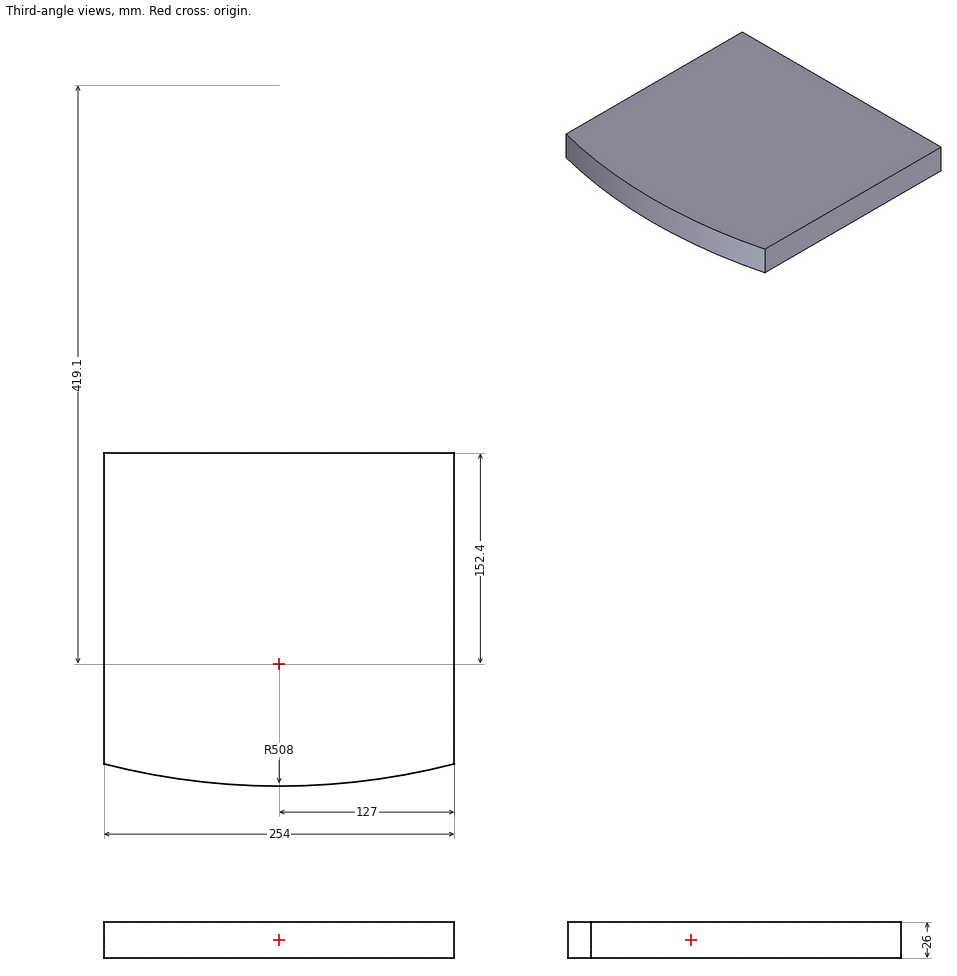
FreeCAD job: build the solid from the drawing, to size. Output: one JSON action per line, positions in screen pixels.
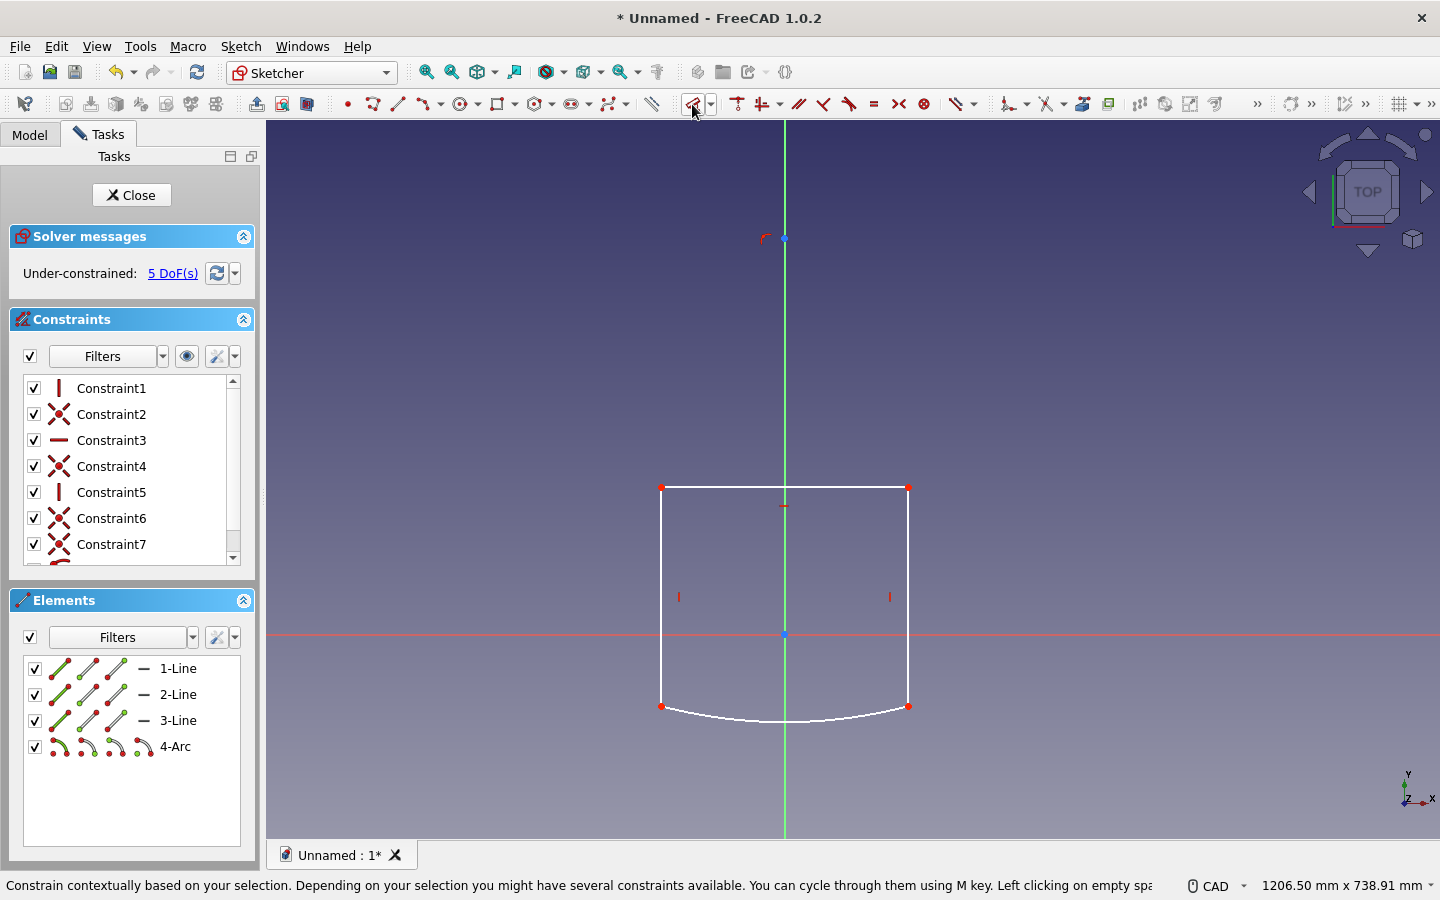
{"action": "left_click", "coordinate": [735, 720]}
{"action": "left_click", "coordinate": [732, 752]}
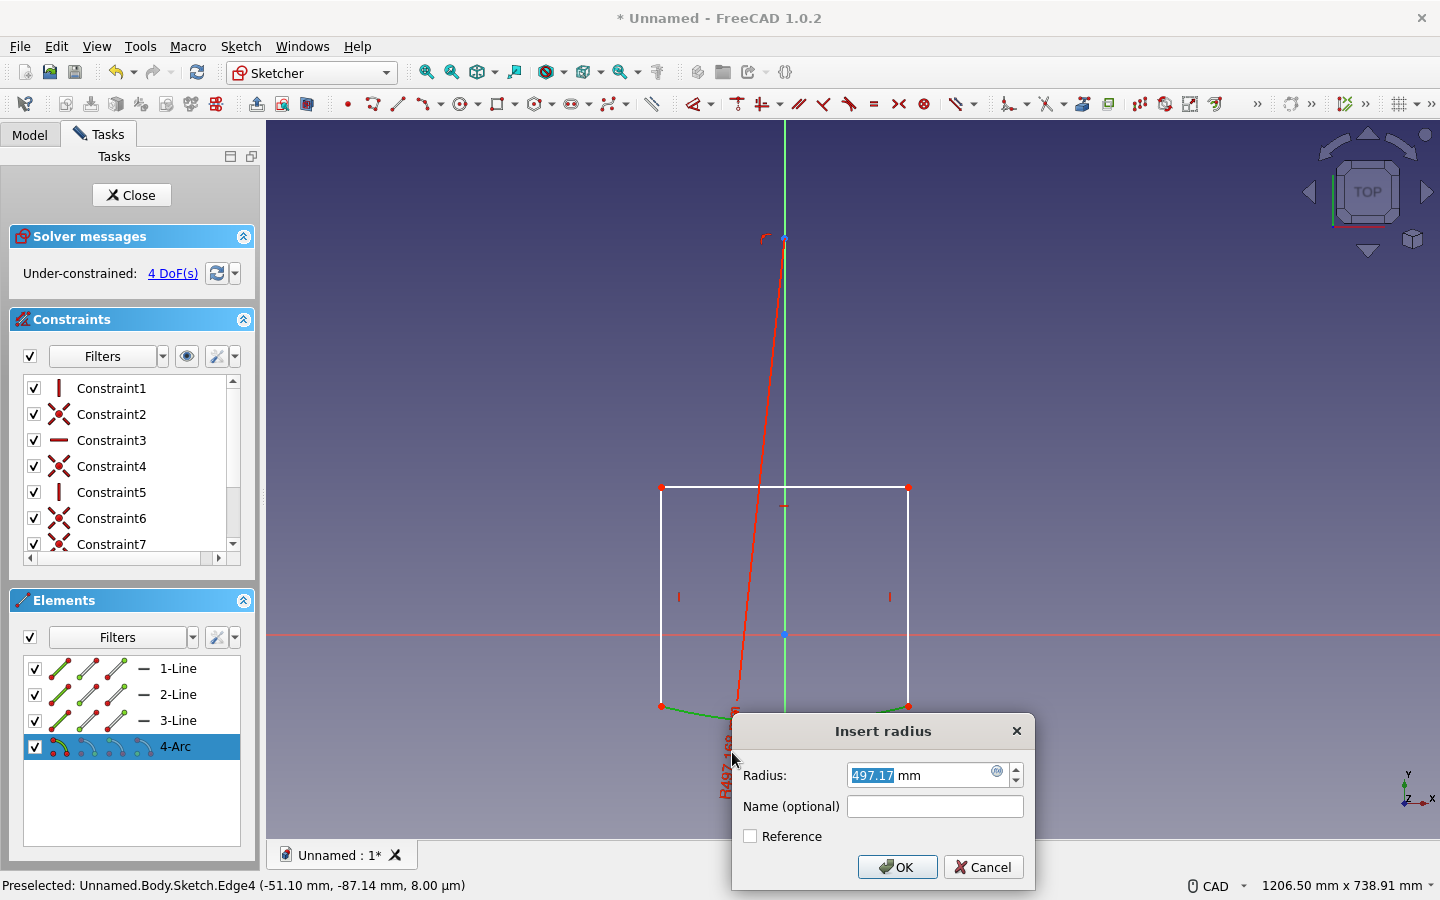
{"action": "type", "text": "508"}
{"action": "key", "text": "Return"}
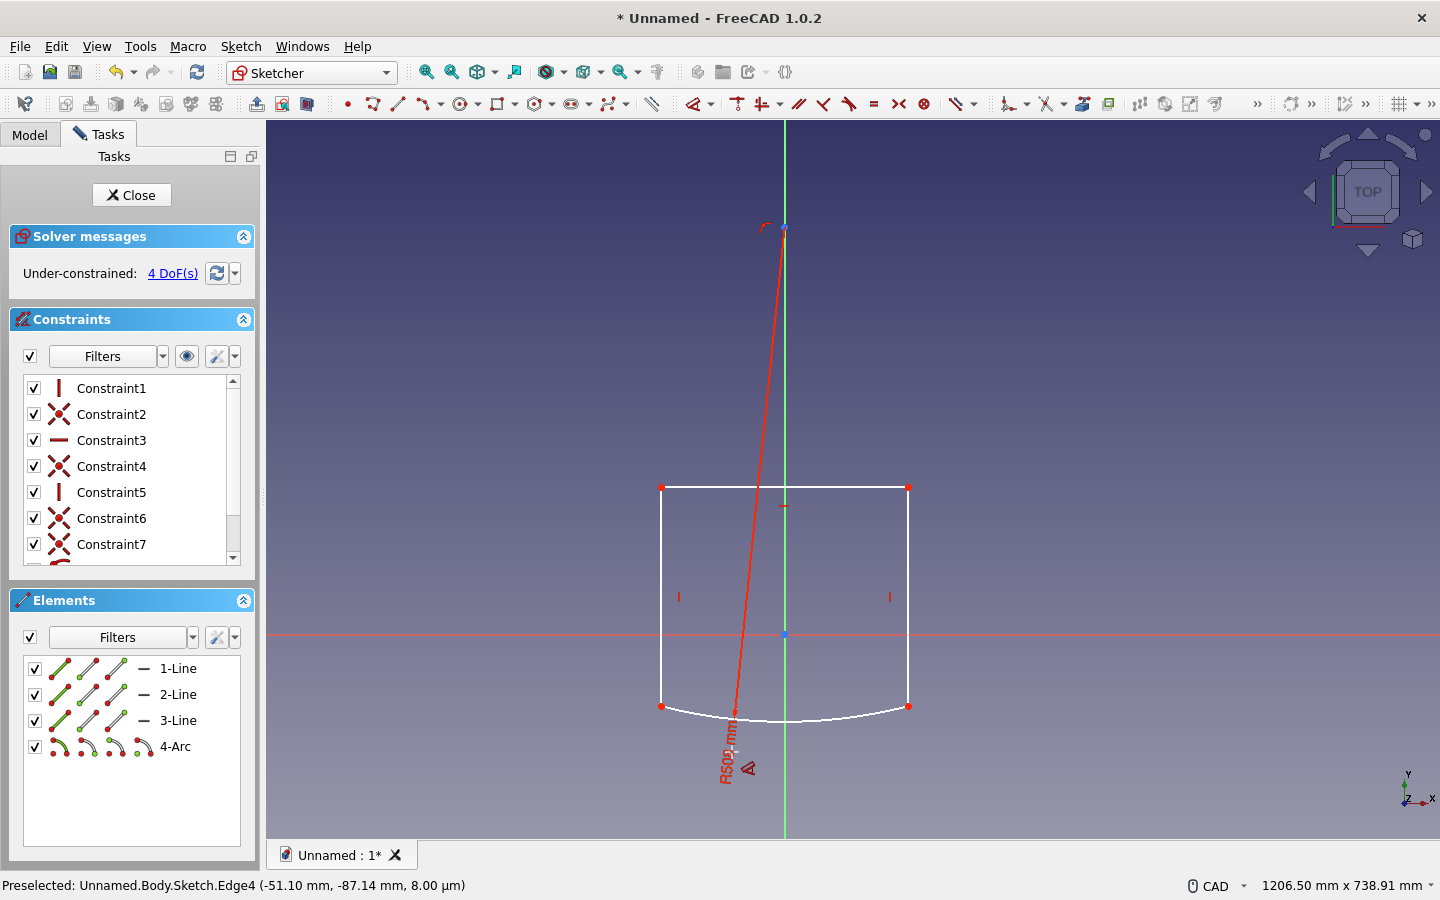
{"action": "left_click", "coordinate": [834, 487]}
{"action": "left_click", "coordinate": [728, 453]}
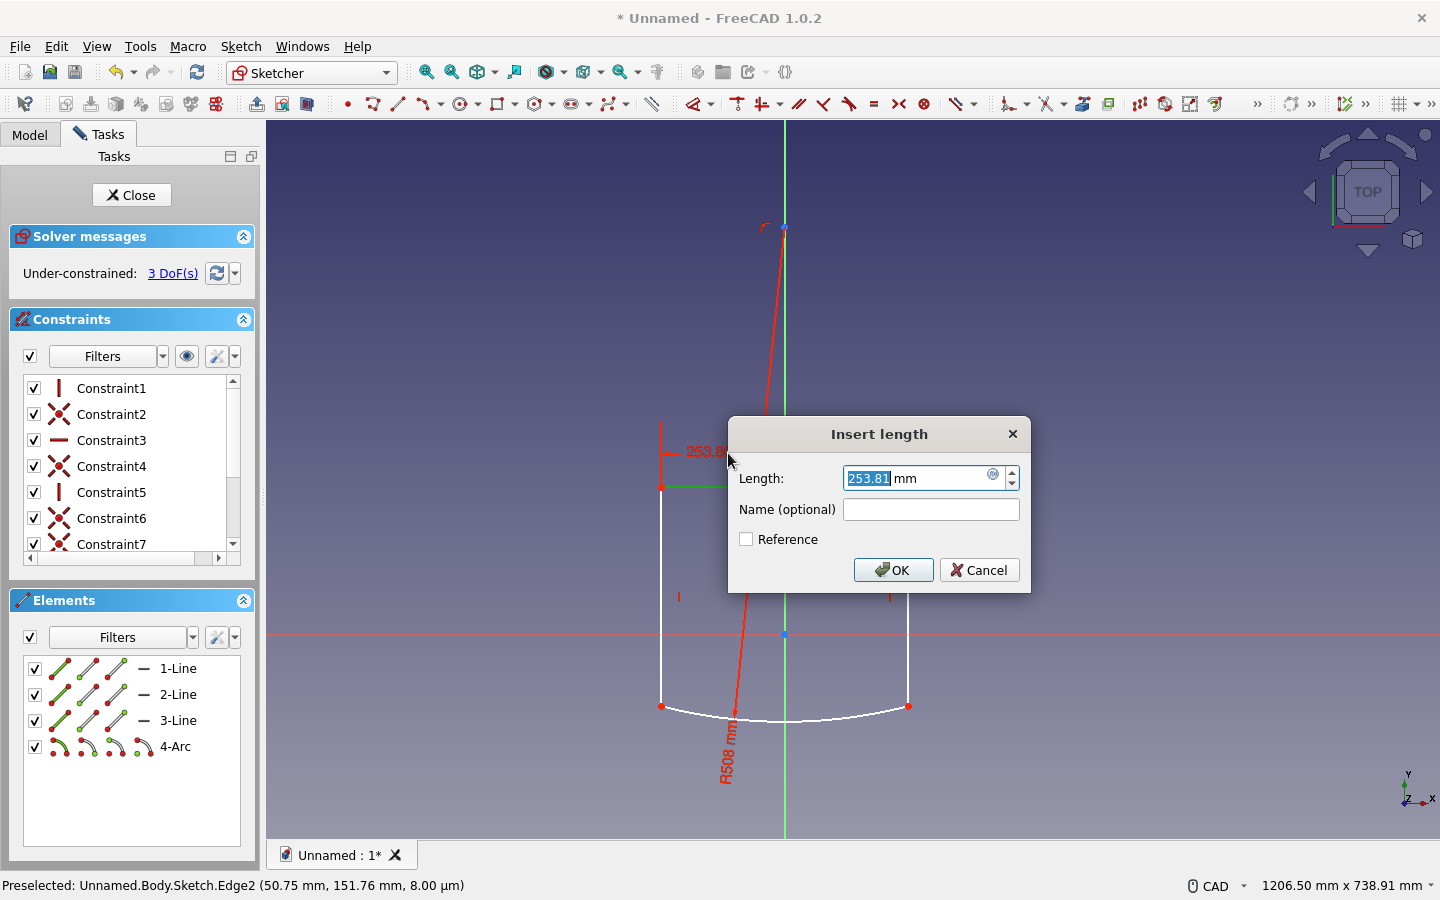
{"action": "type", "text": "254"}
{"action": "key", "text": "Return"}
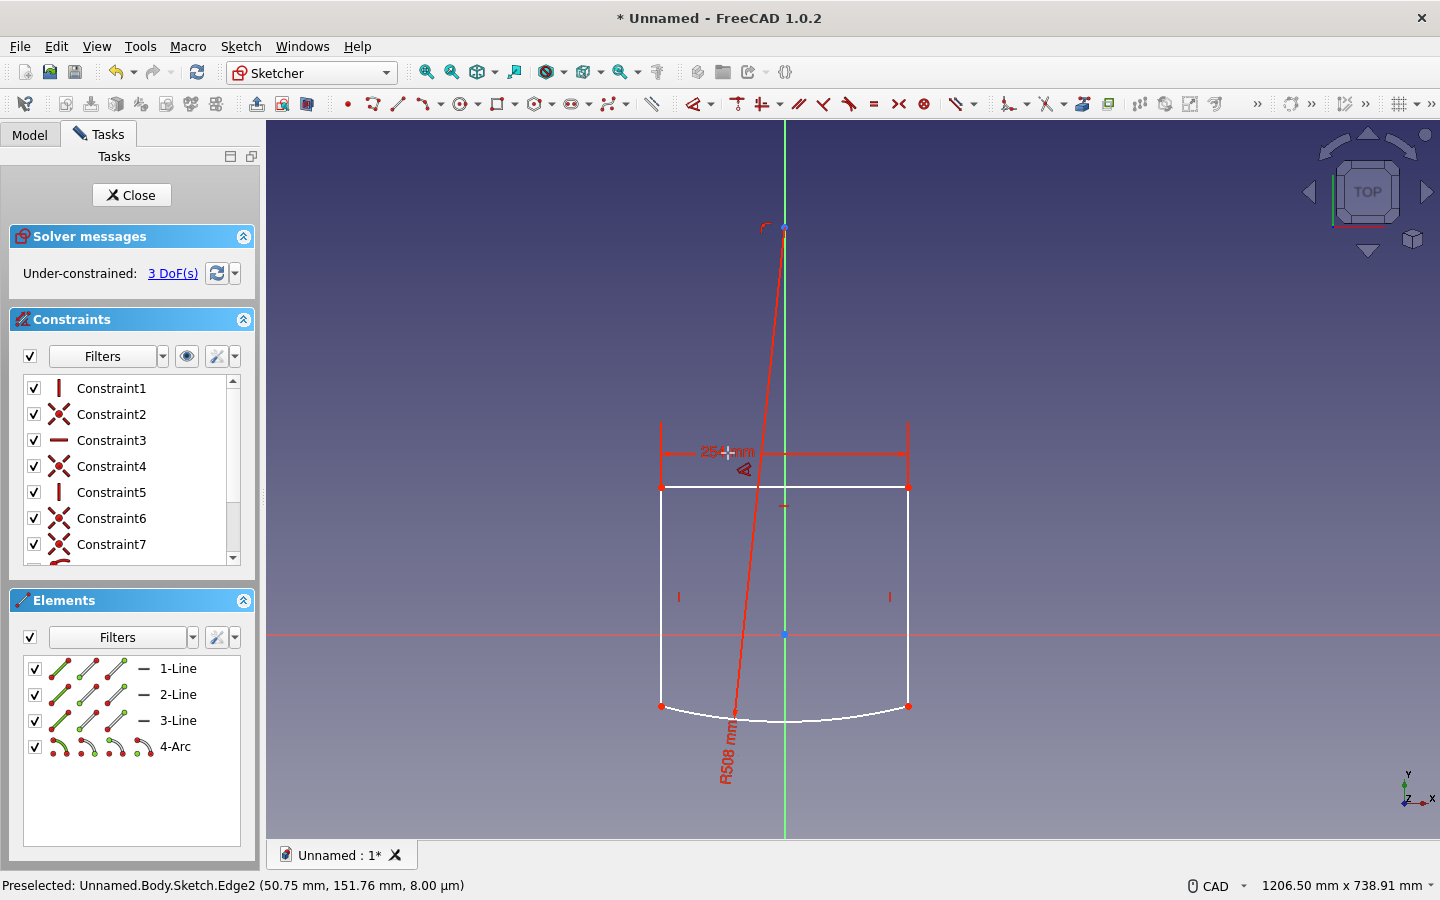
{"action": "left_click", "coordinate": [908, 706]}
{"action": "left_click", "coordinate": [846, 740]}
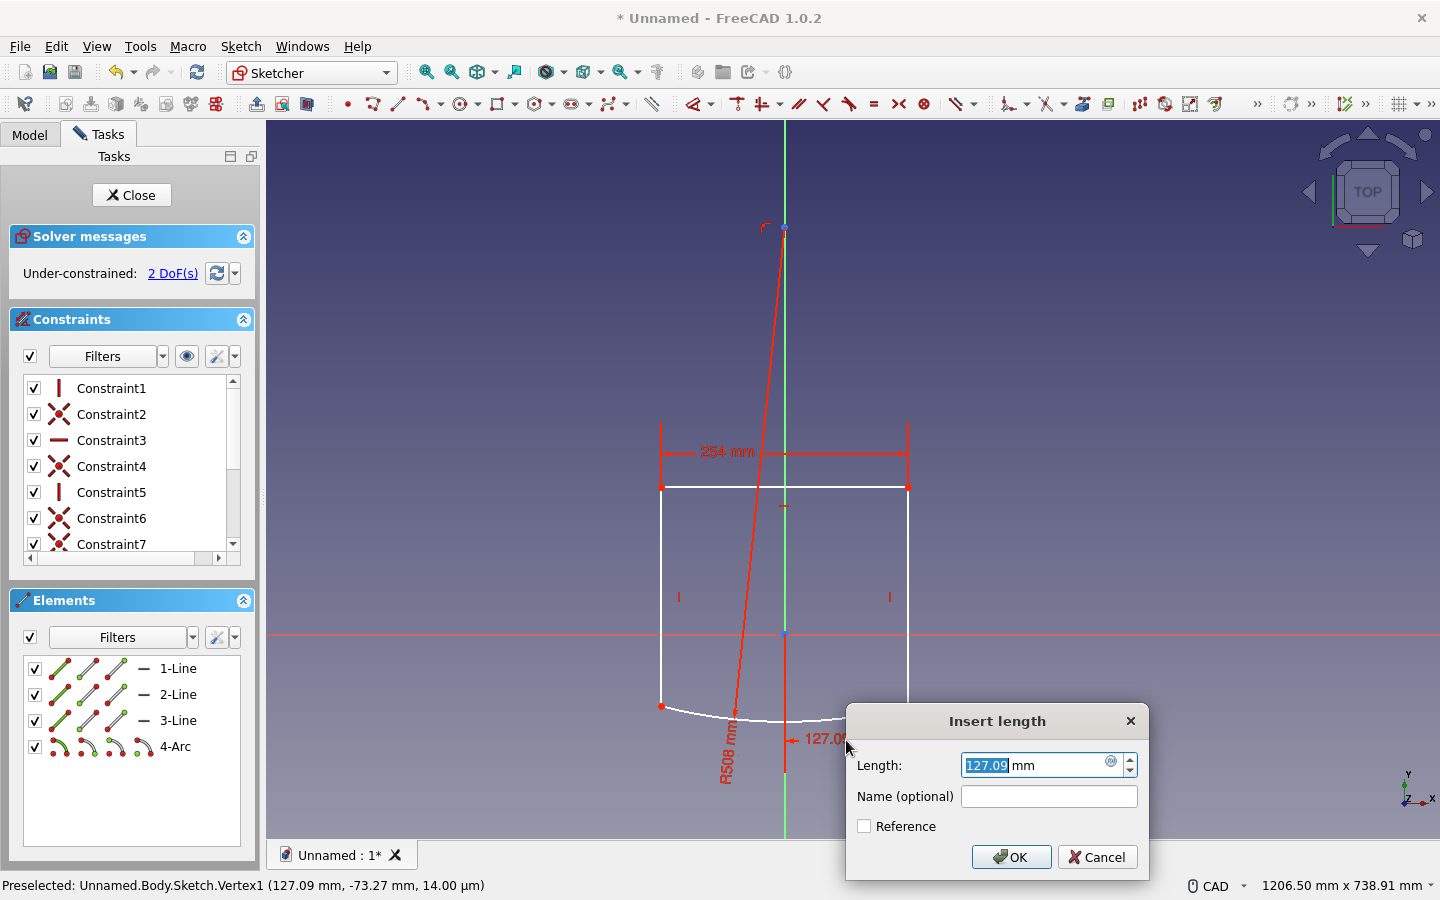
{"action": "type", "text": "127"}
{"action": "key", "text": "Return"}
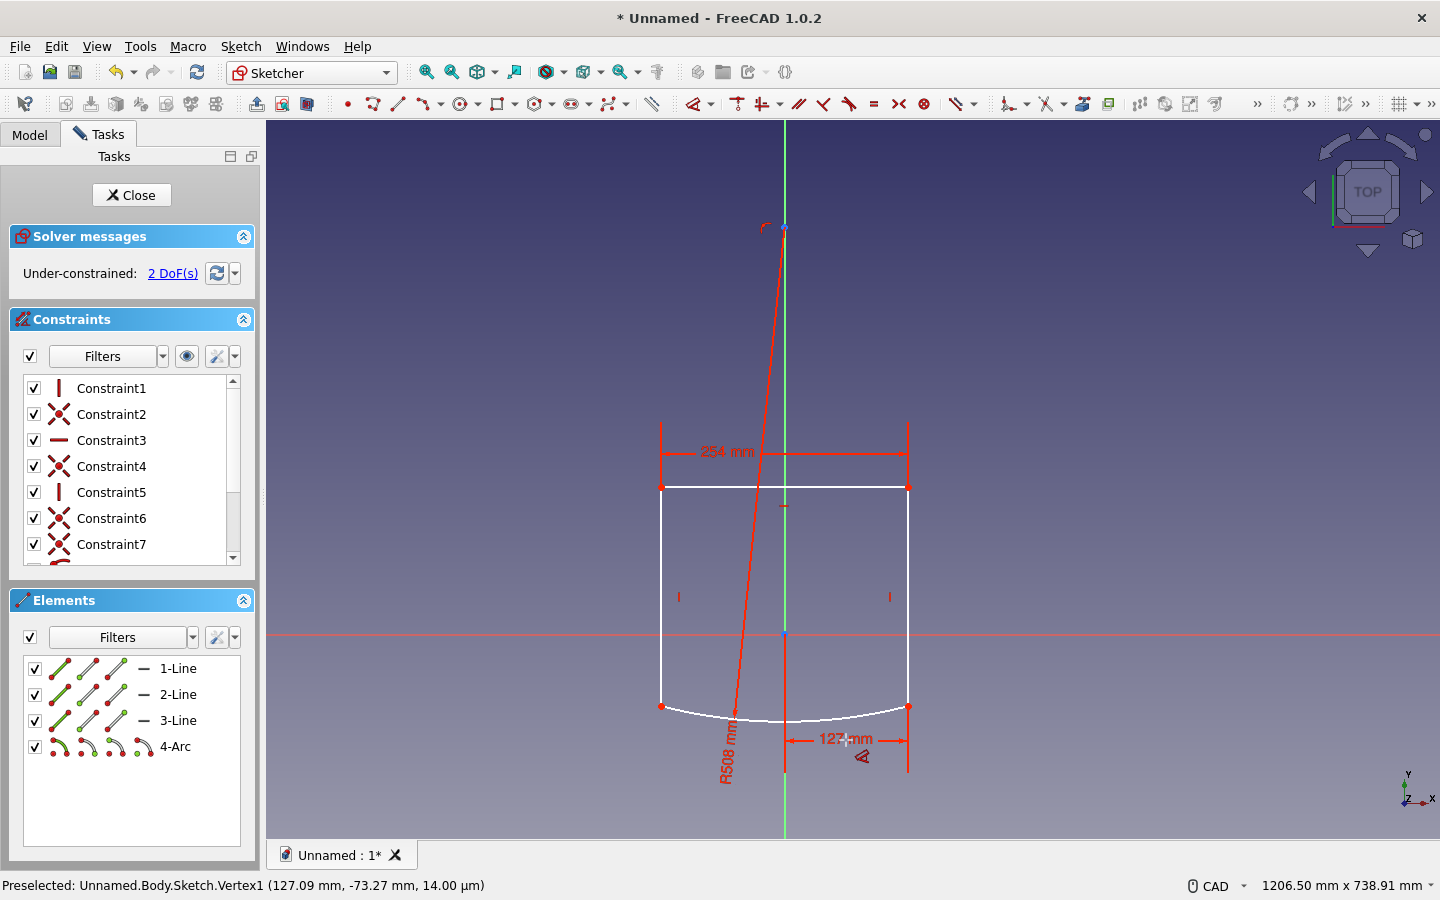
{"action": "left_click", "coordinate": [908, 487]}
{"action": "left_click", "coordinate": [942, 561]}